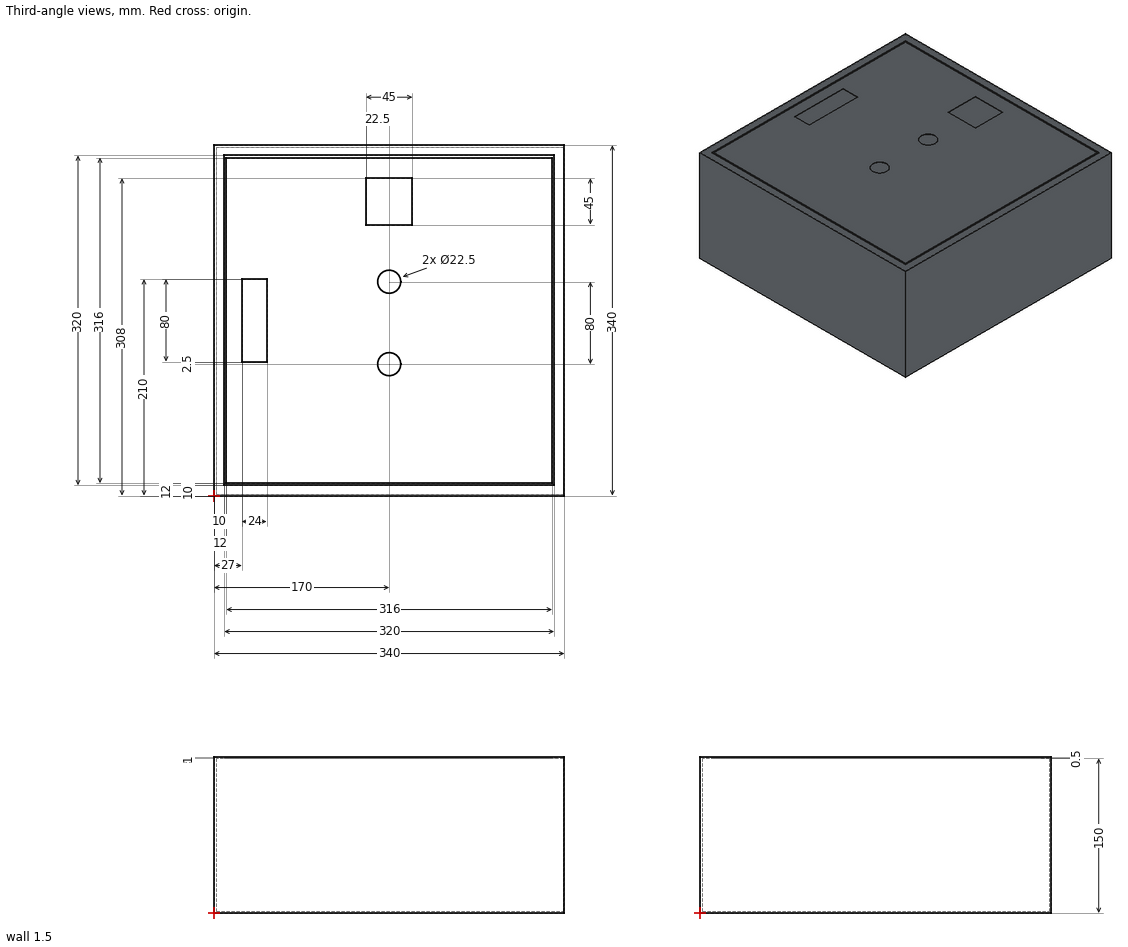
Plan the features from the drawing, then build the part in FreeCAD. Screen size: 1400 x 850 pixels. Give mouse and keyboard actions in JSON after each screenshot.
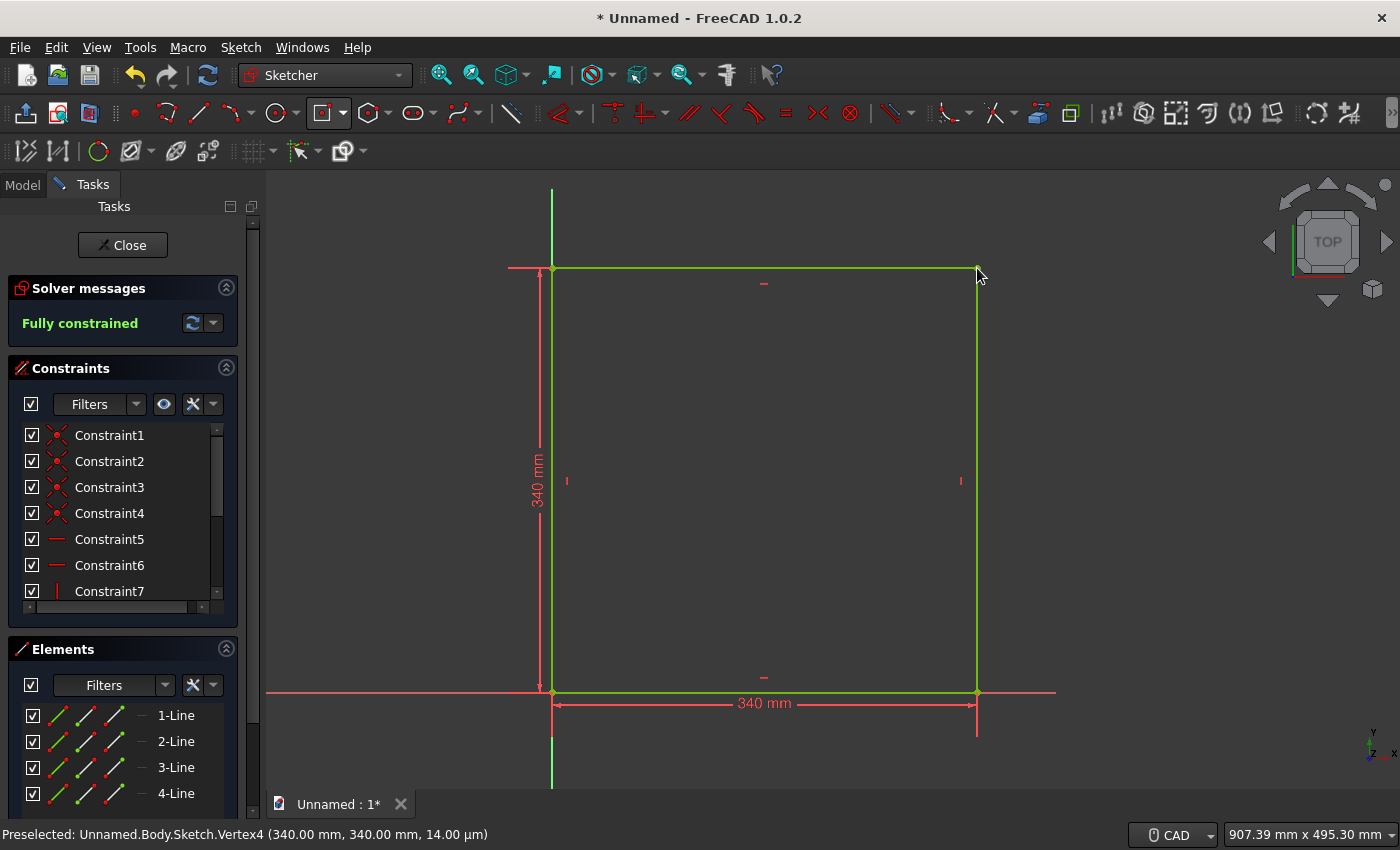
{"action": "left_click", "coordinate": [123, 245]}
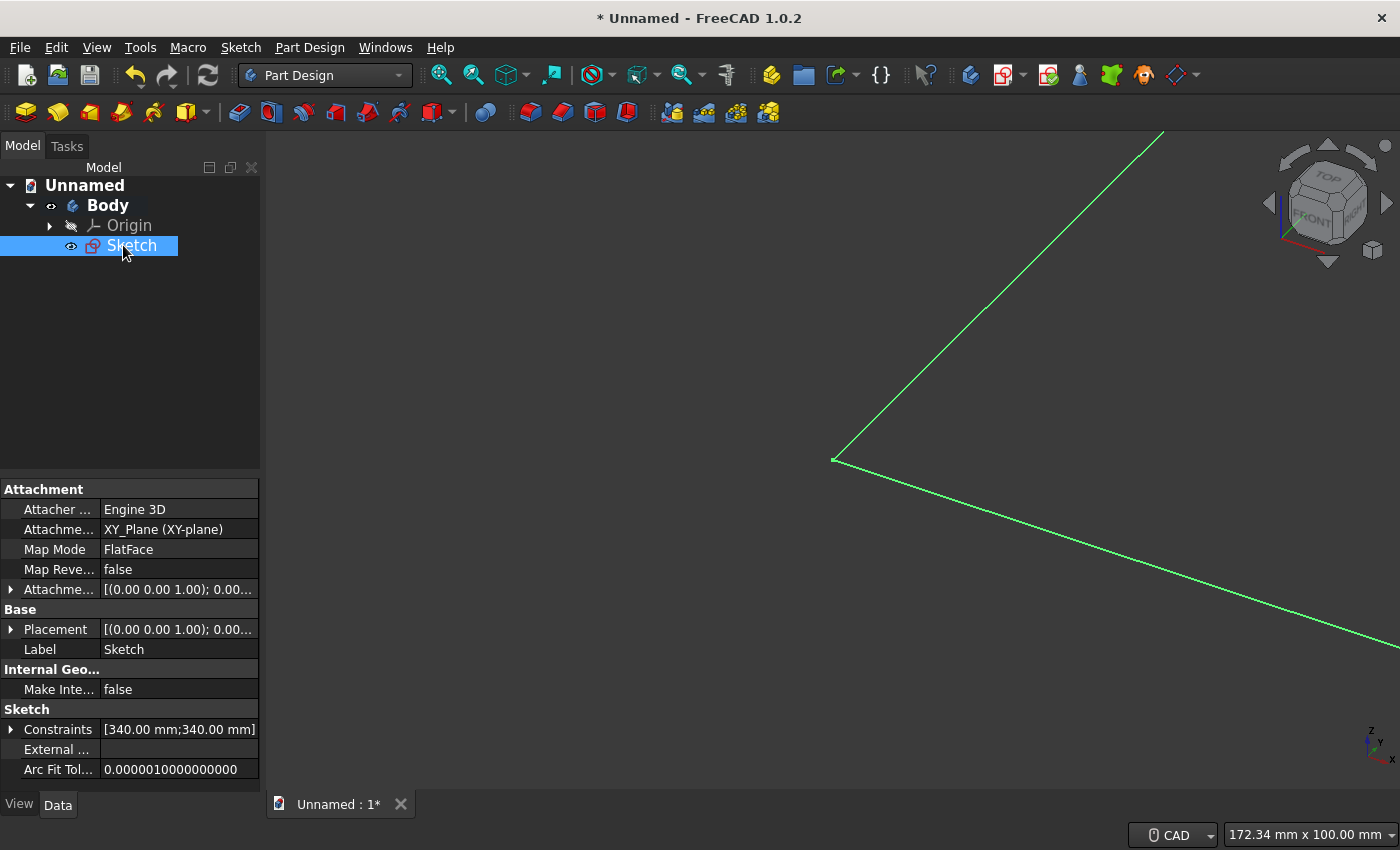
{"action": "left_click", "coordinate": [26, 112]}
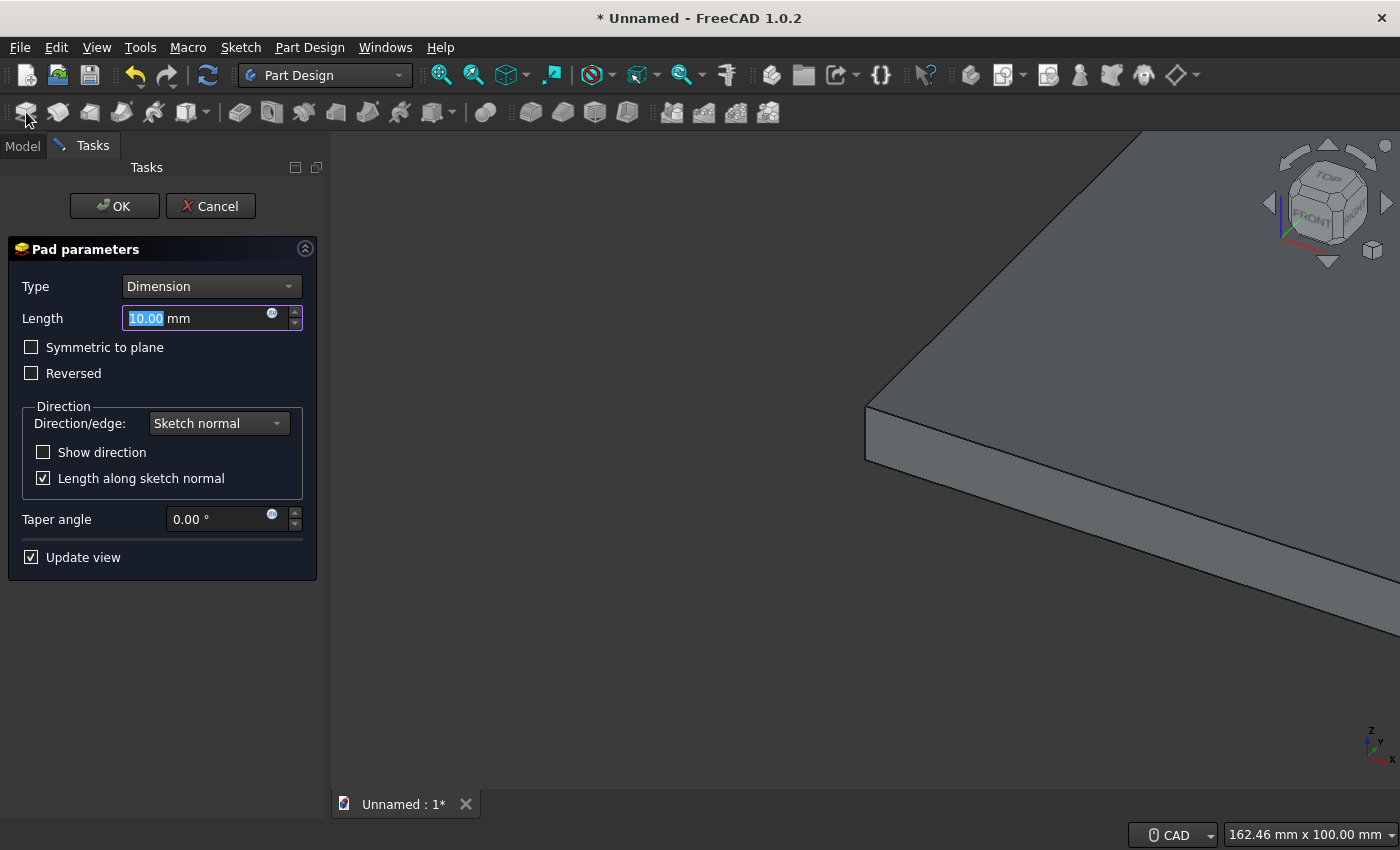
{"action": "type", "text": "150"}
{"action": "key", "text": "Tab"}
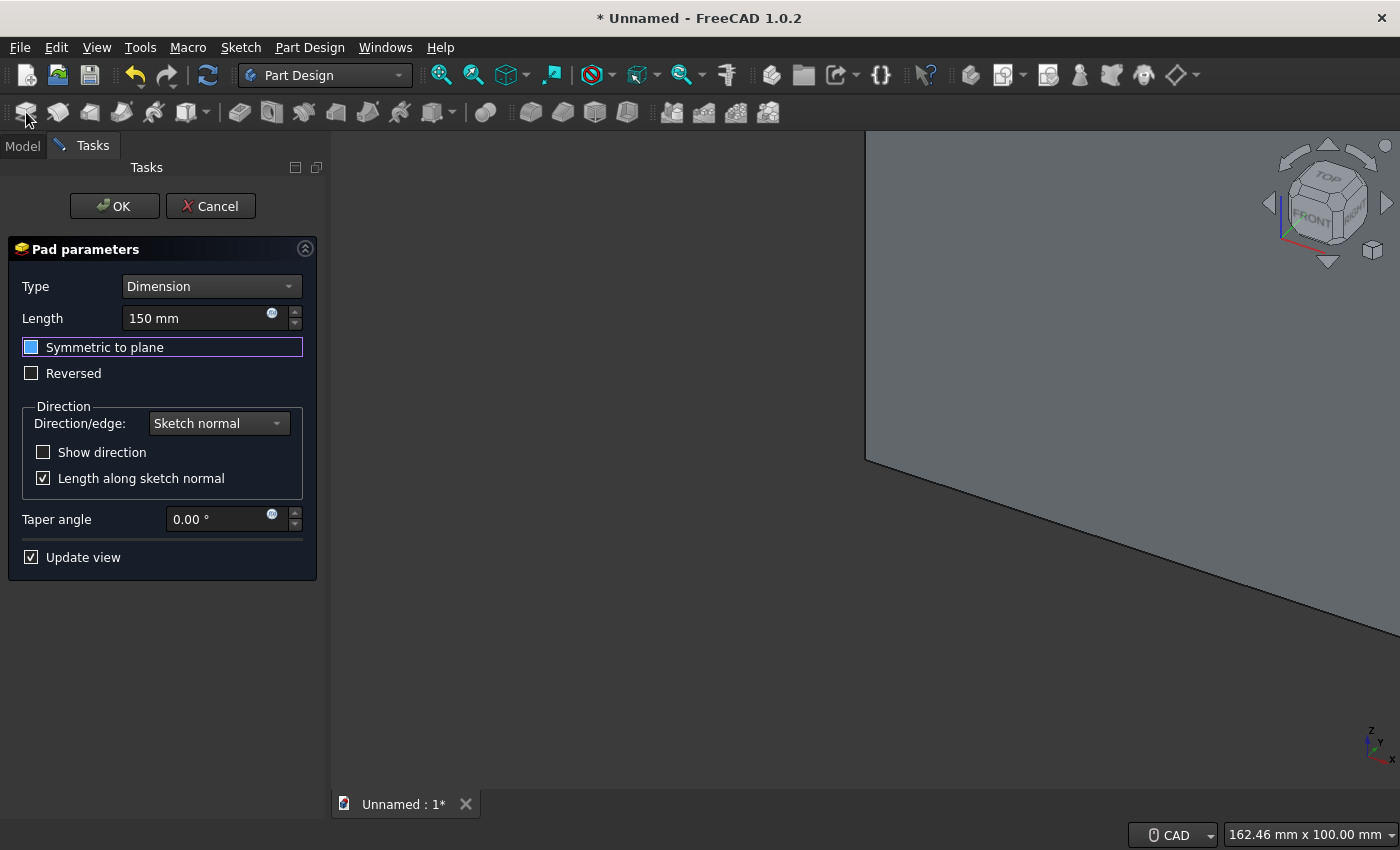
{"action": "left_click", "coordinate": [115, 206]}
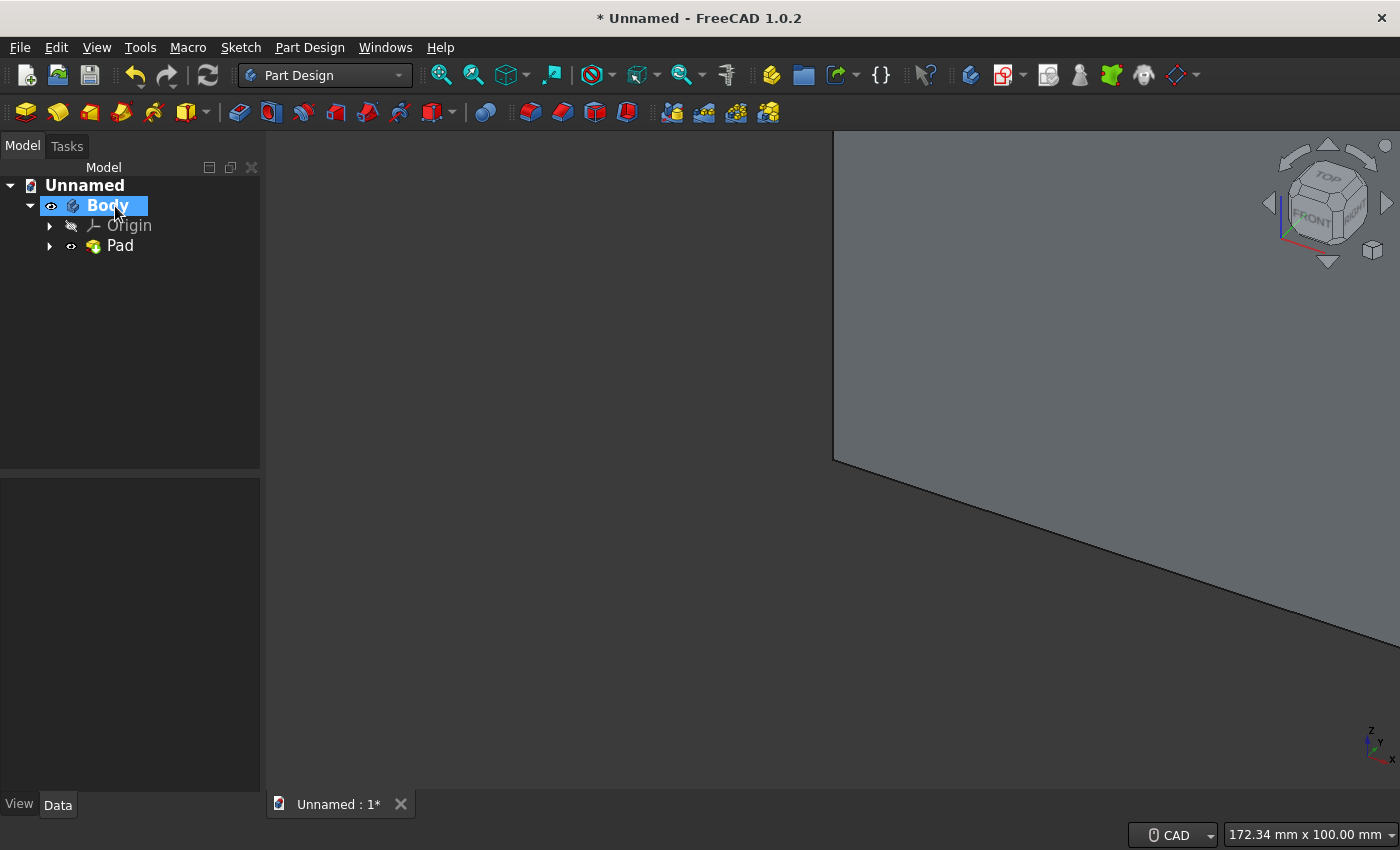
{"action": "left_click", "coordinate": [442, 76]}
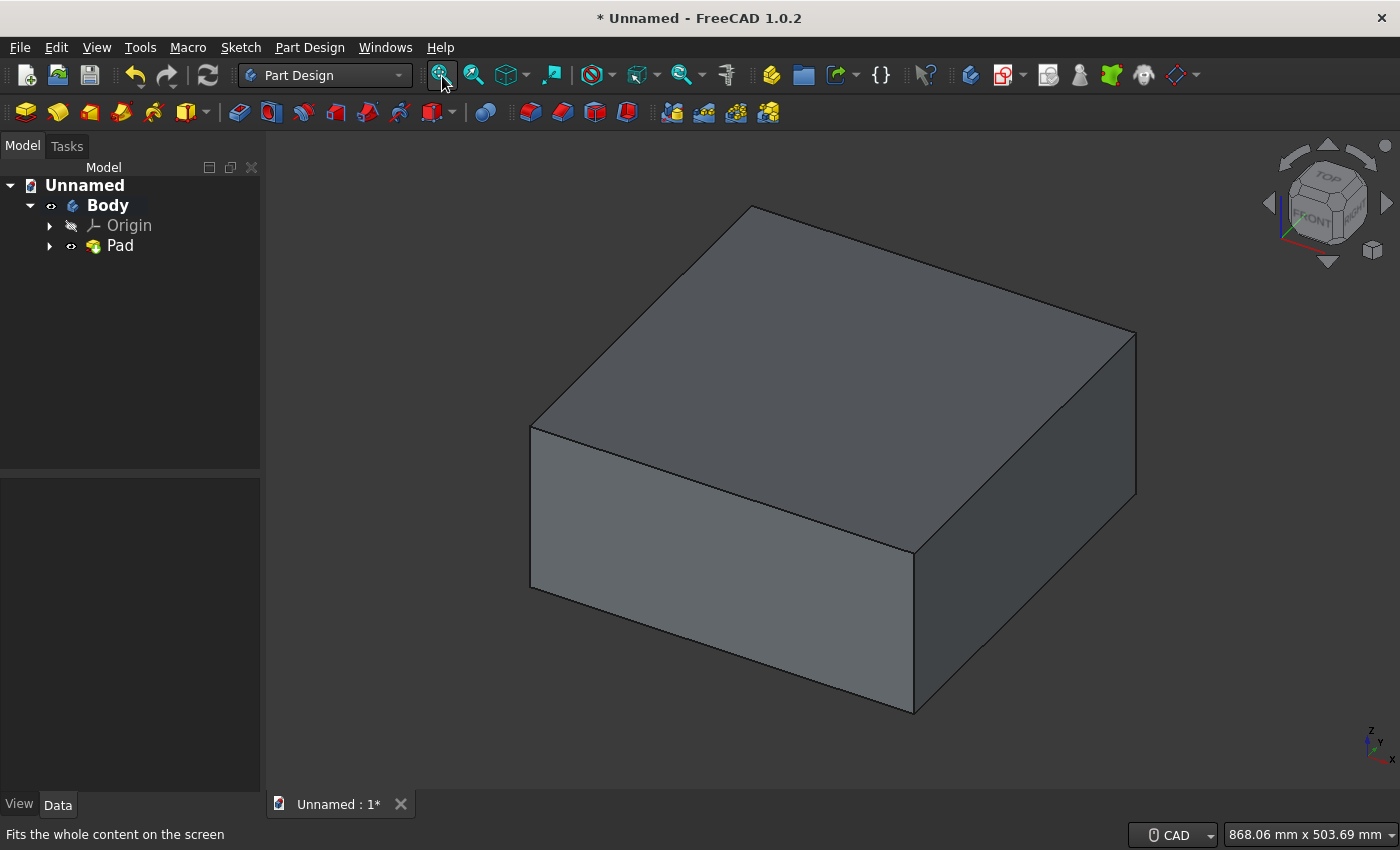
{"action": "left_click", "coordinate": [833, 379]}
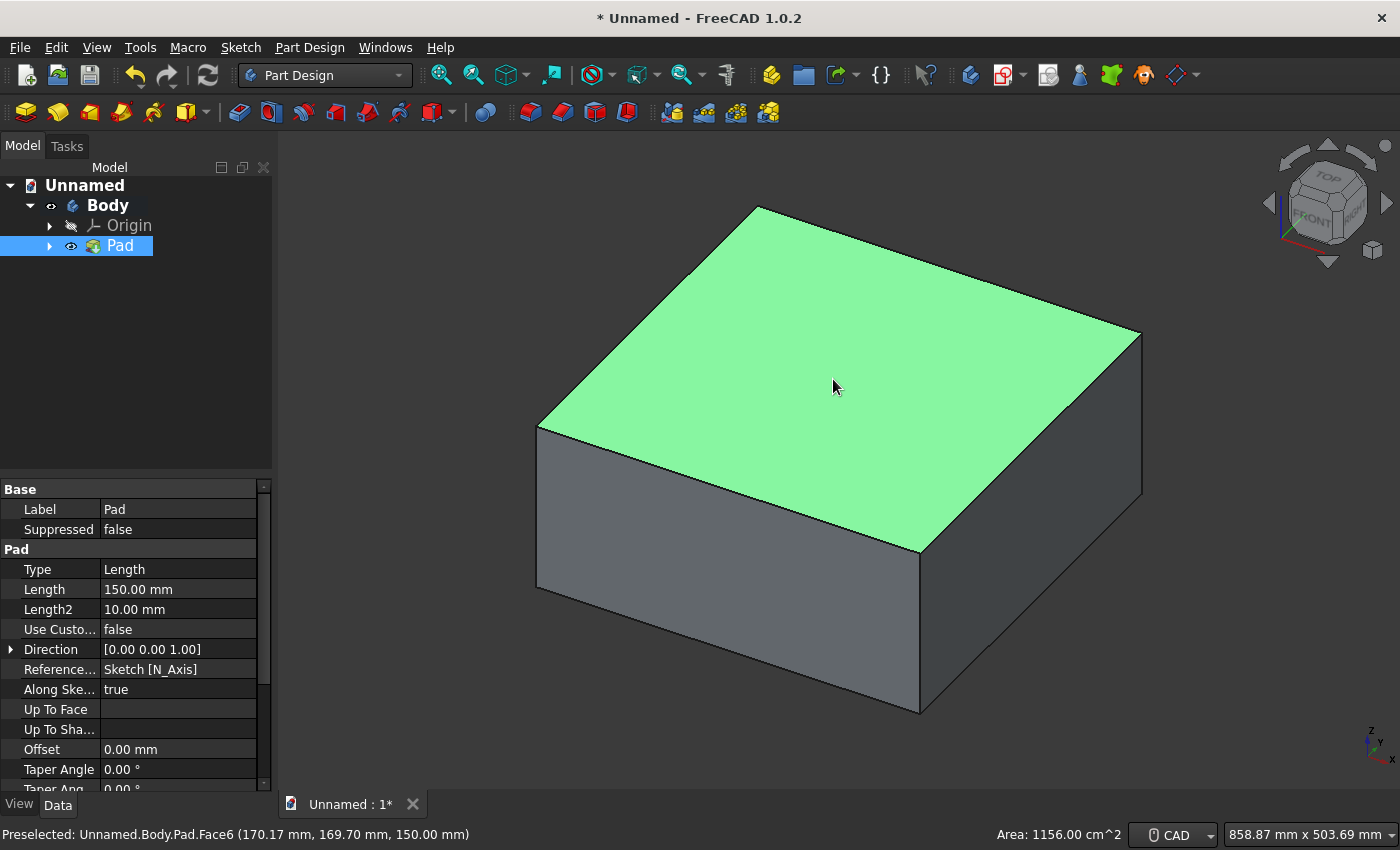
{"action": "left_click", "coordinate": [628, 112]}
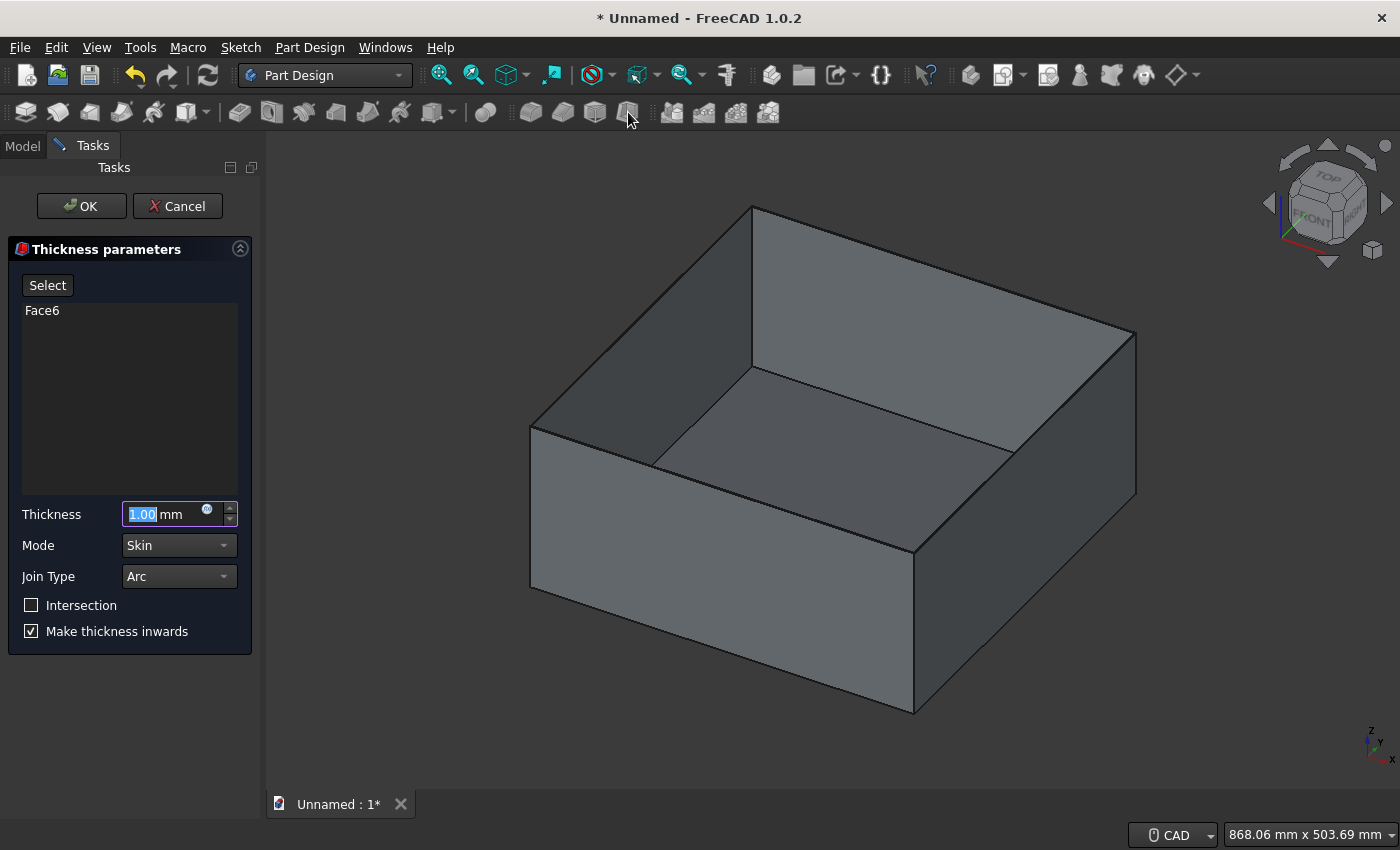
{"action": "type", "text": "1.5"}
{"action": "key", "text": "Tab"}